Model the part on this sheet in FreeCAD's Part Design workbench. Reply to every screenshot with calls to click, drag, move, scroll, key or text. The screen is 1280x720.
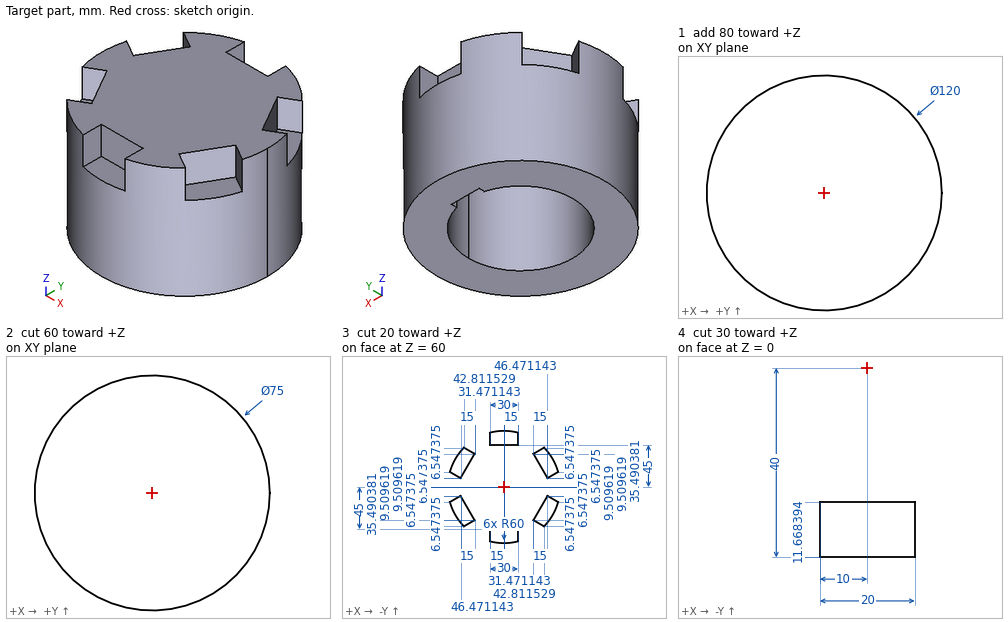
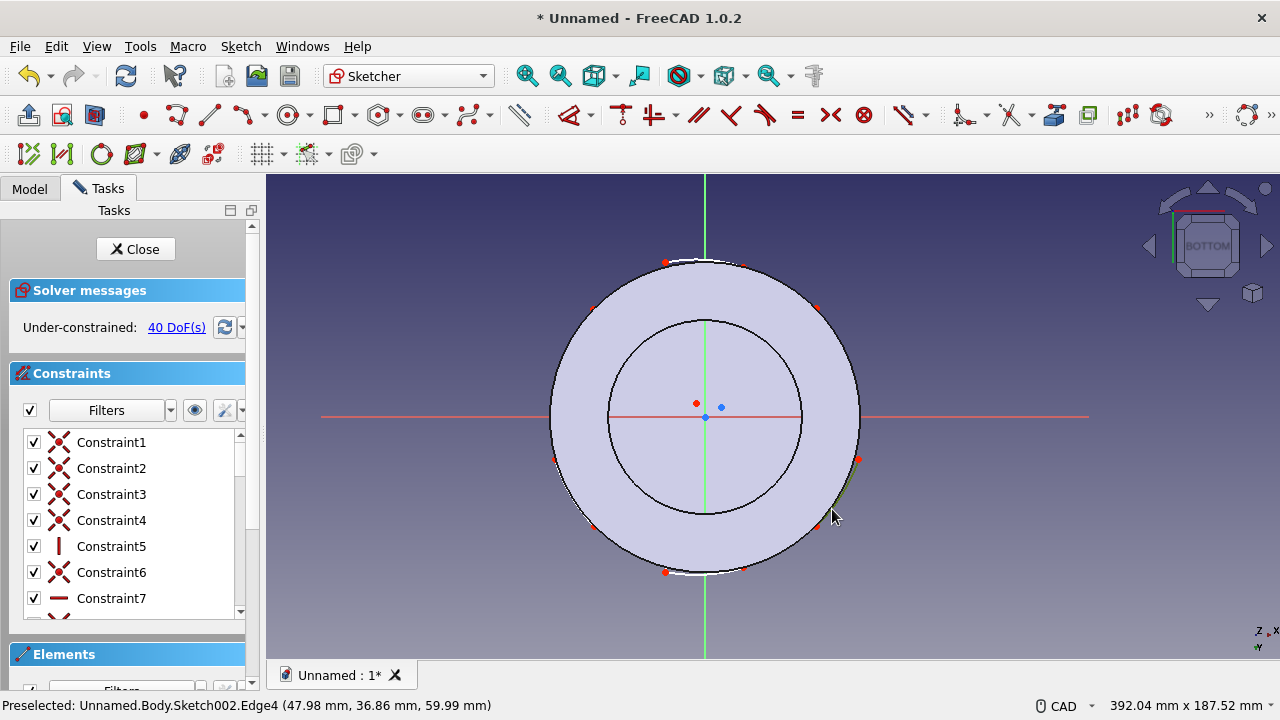
click(563, 482)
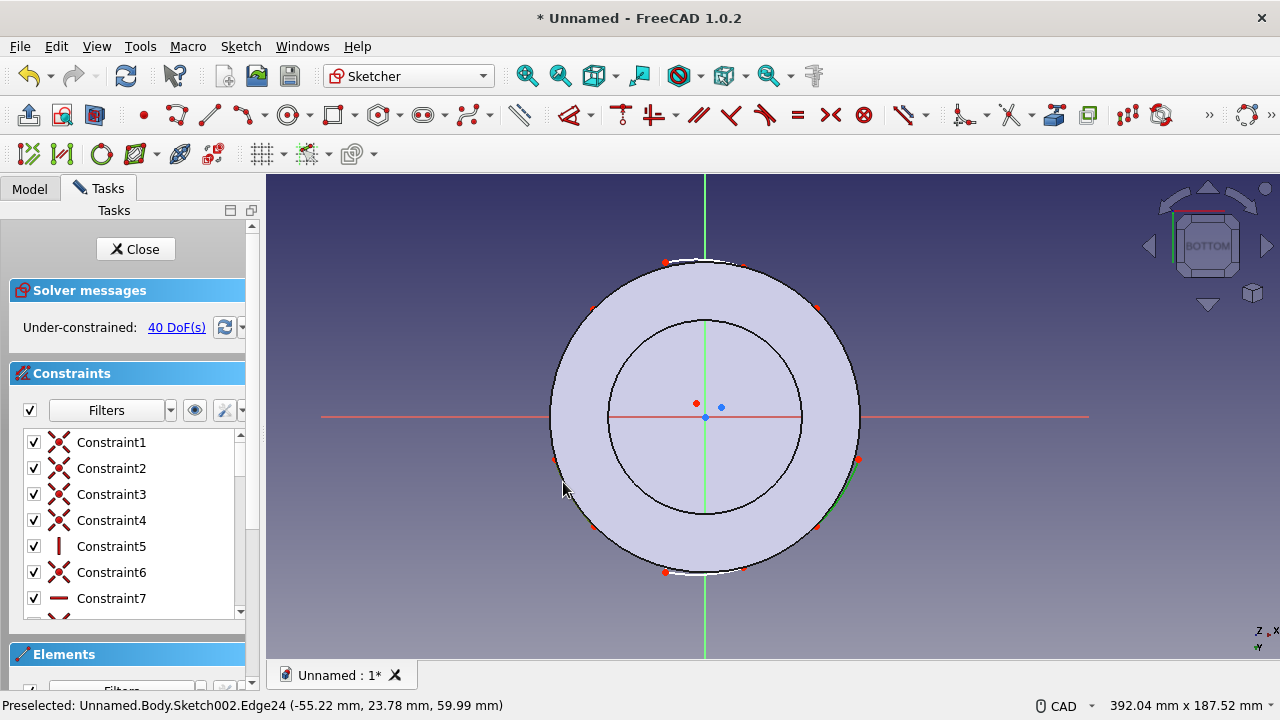
click(621, 116)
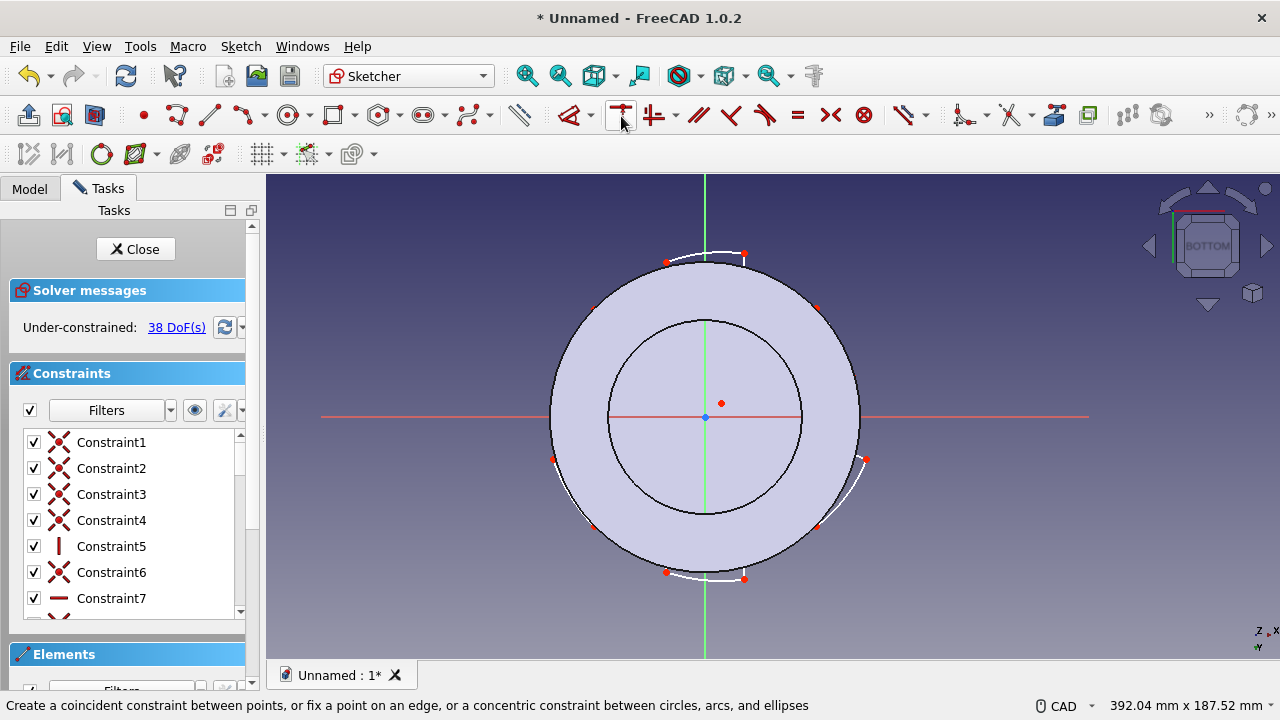
drag(695, 393, 732, 427)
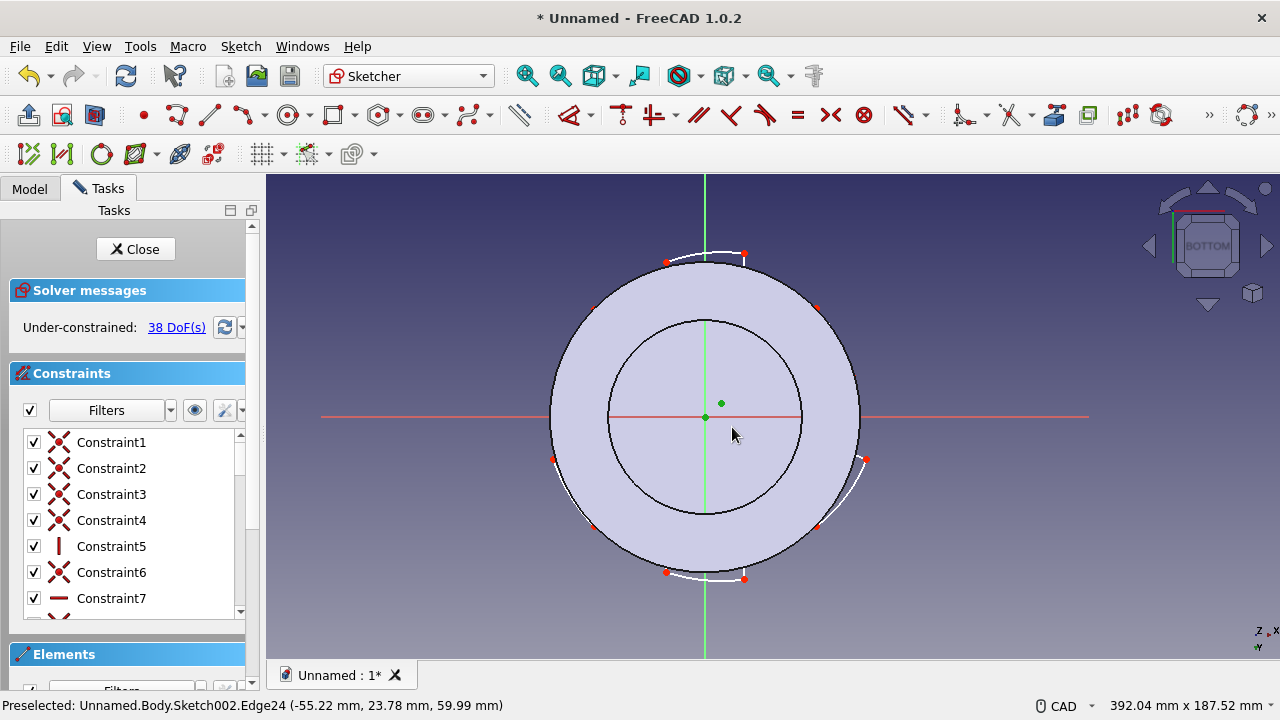
click(621, 116)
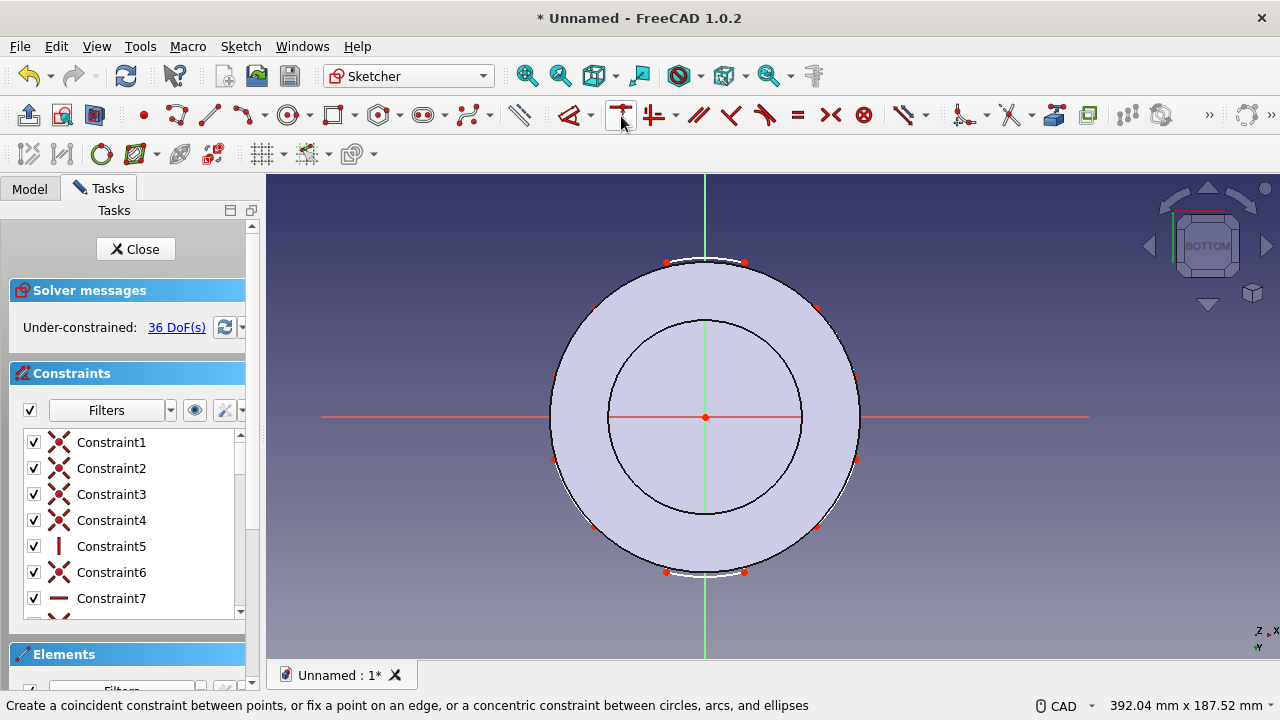
click(831, 509)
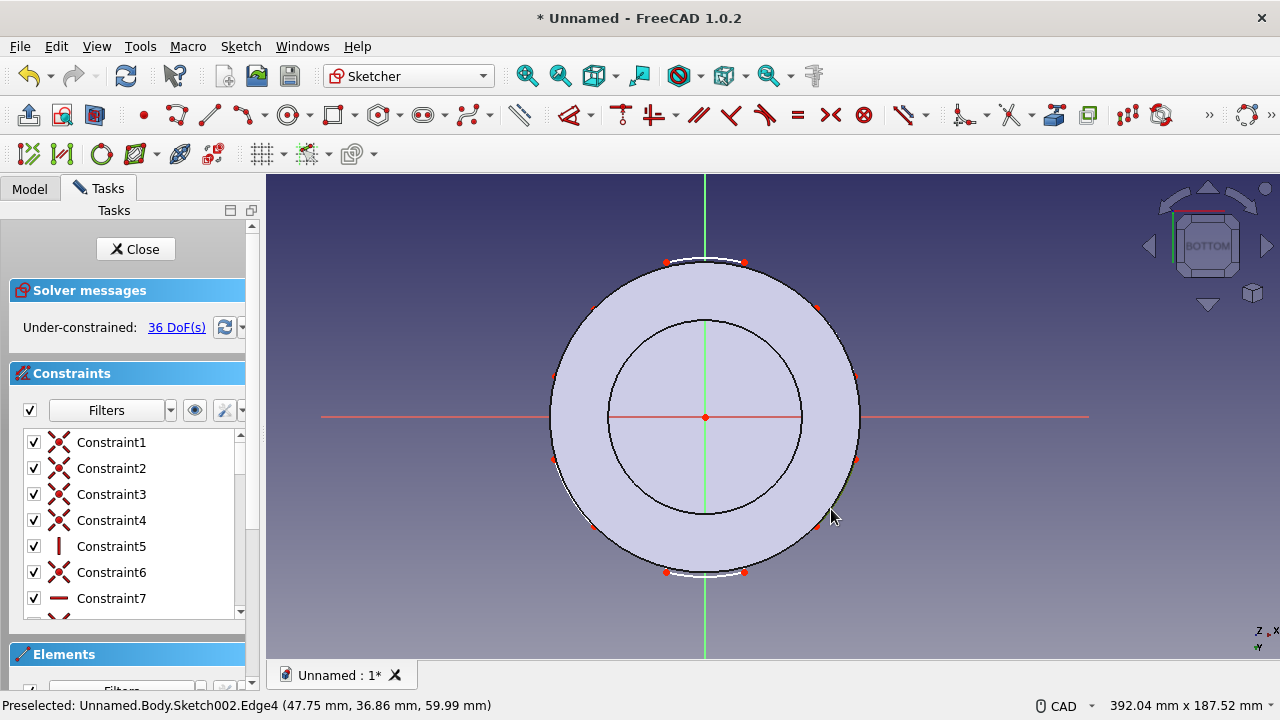
click(689, 576)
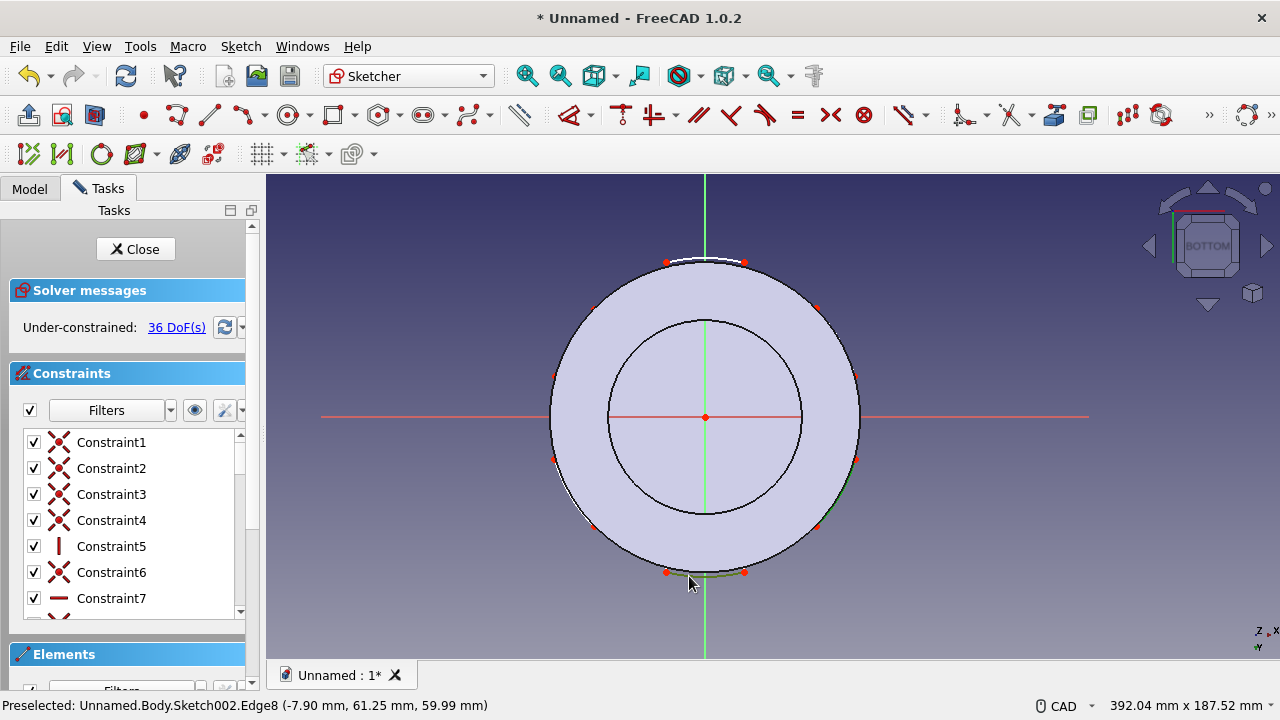
click(847, 355)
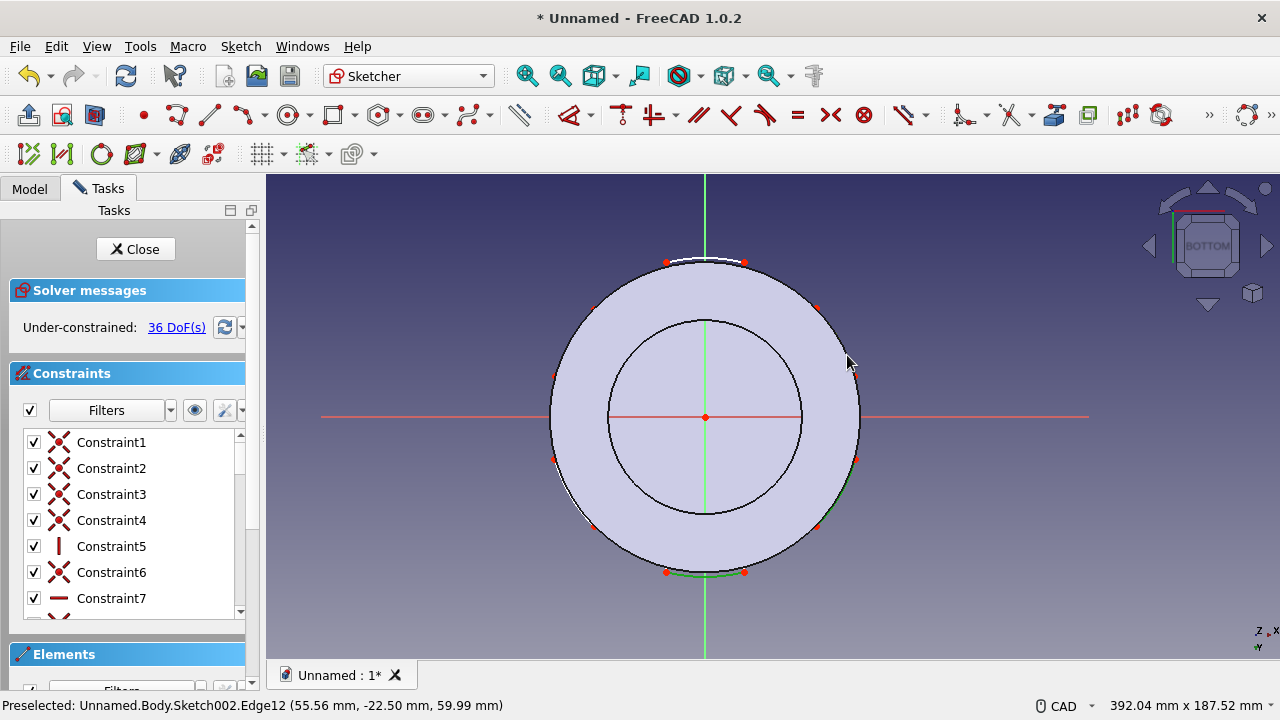
click(721, 259)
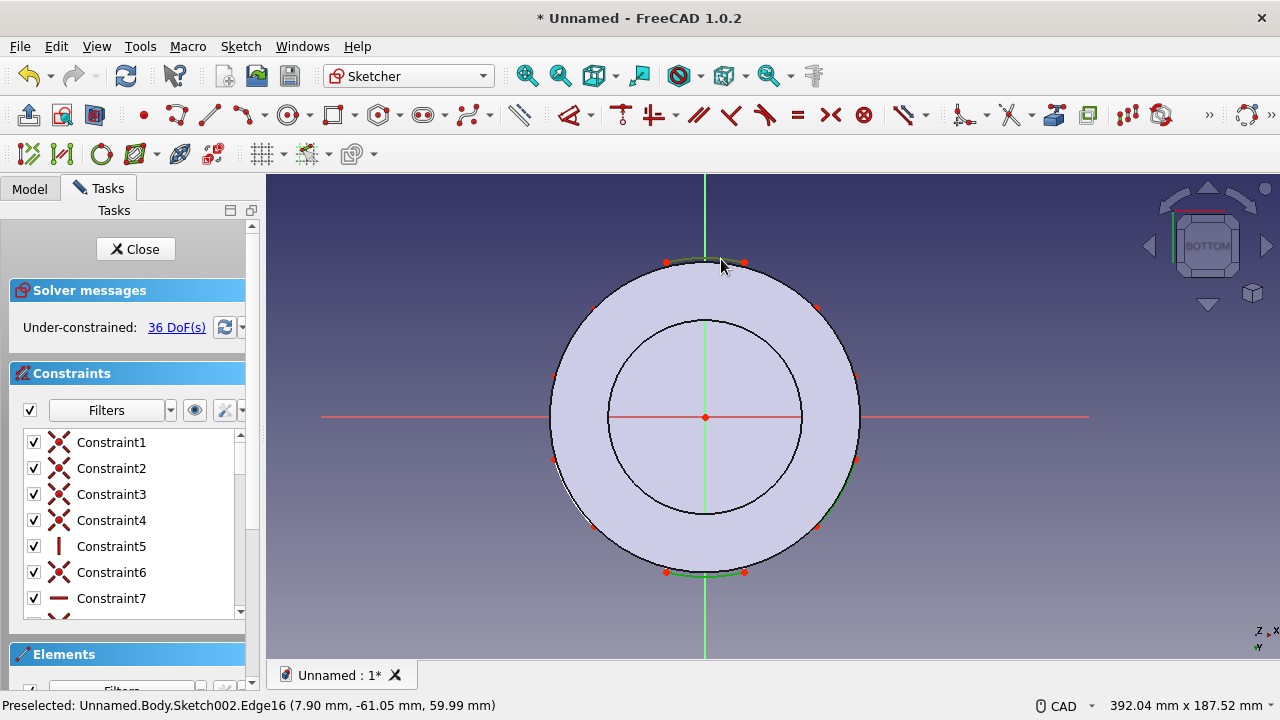
click(579, 328)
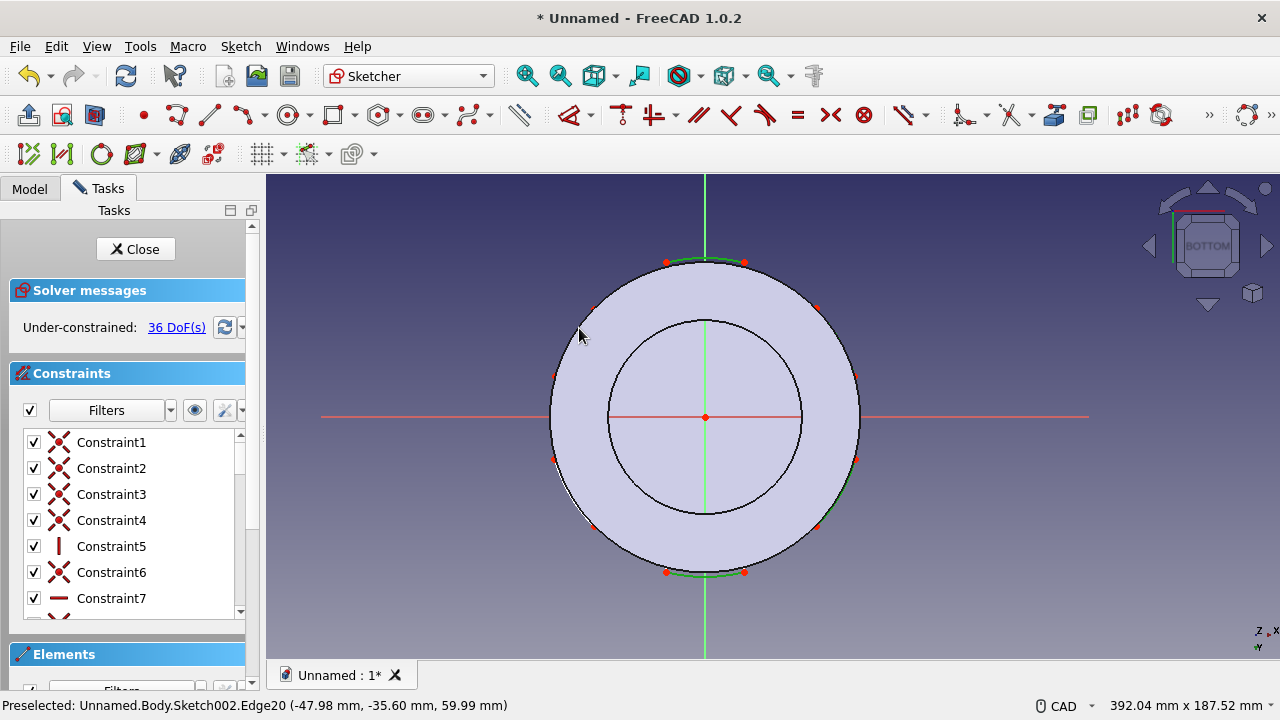
click(563, 482)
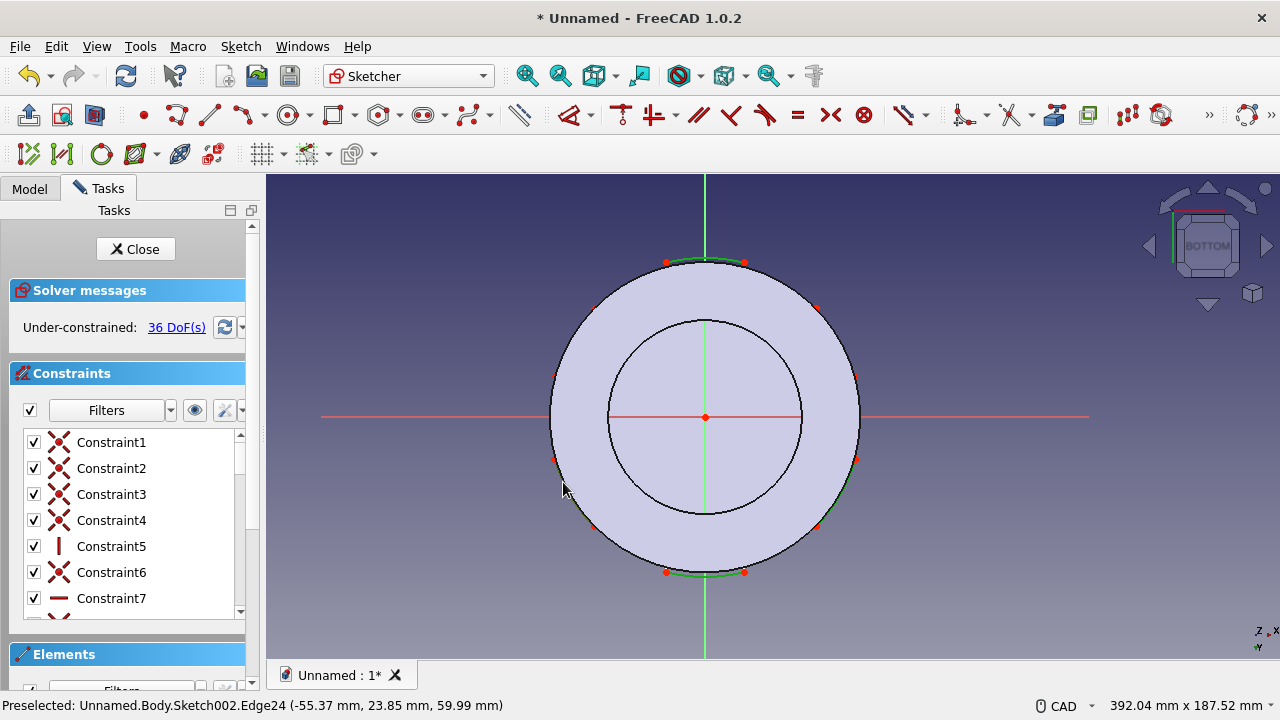
click(798, 116)